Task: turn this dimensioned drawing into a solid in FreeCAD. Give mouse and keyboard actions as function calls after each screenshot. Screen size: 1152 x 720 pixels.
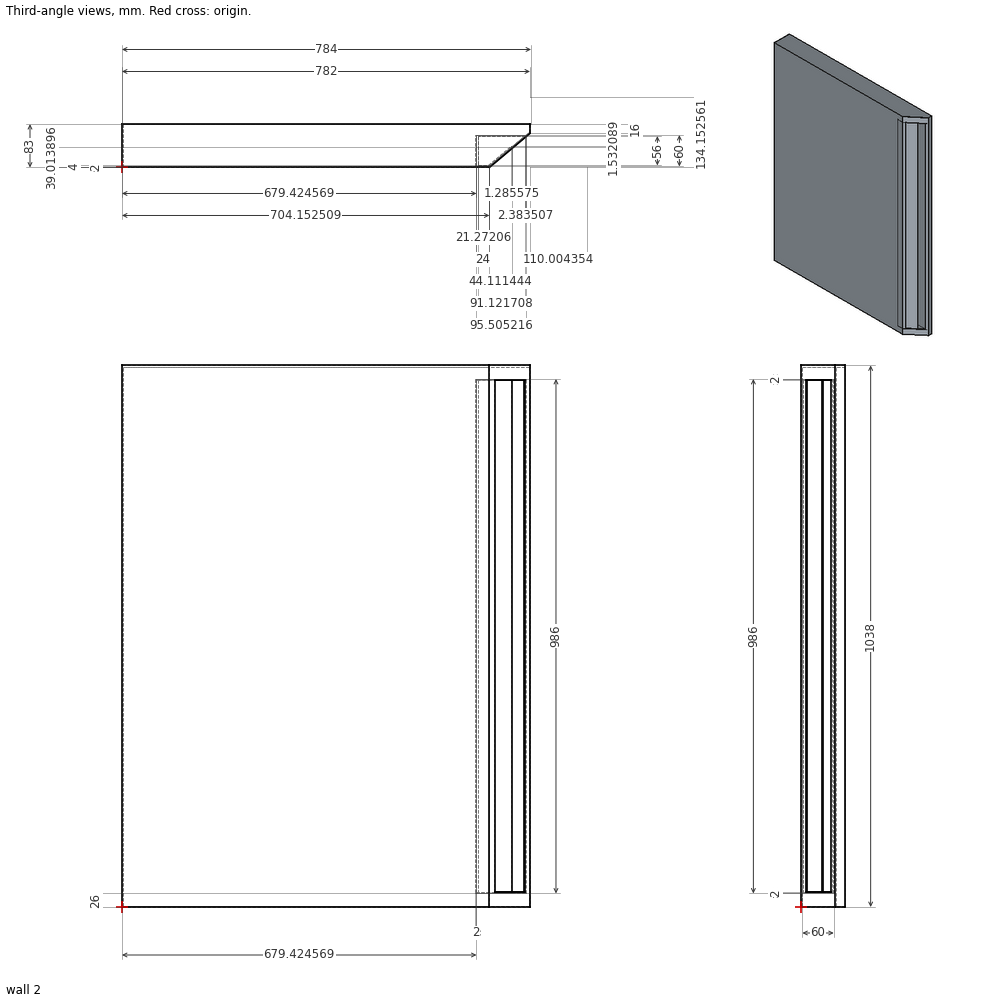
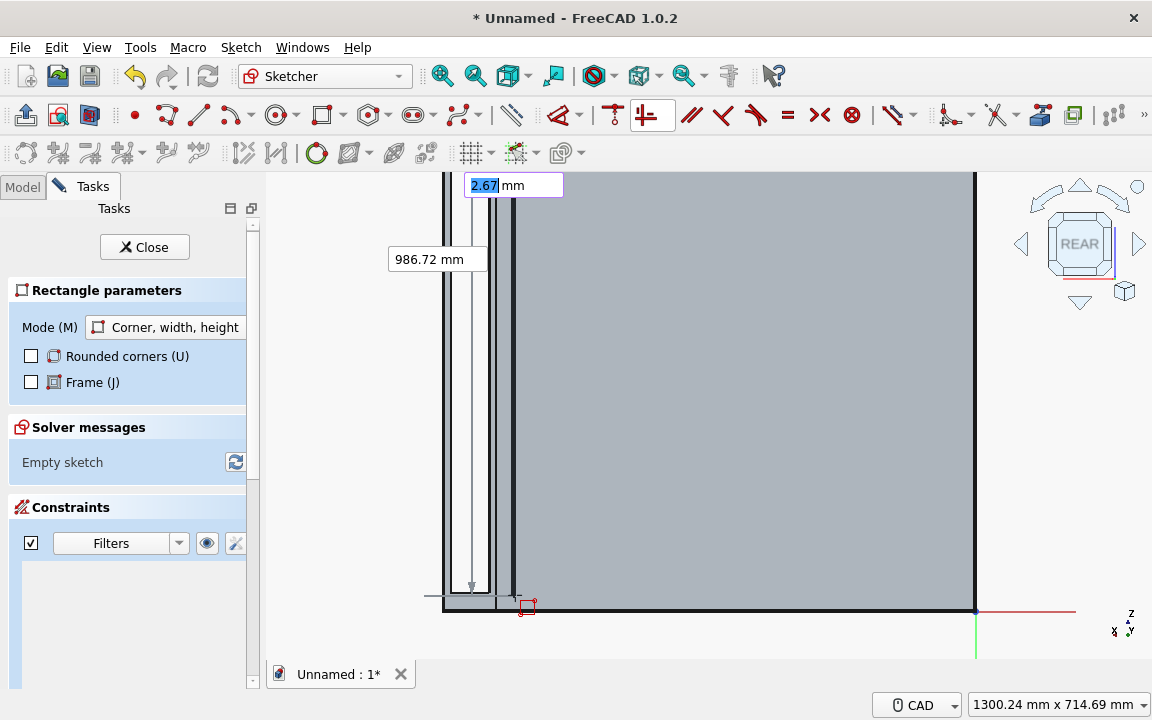
click(514, 594)
key(Escape)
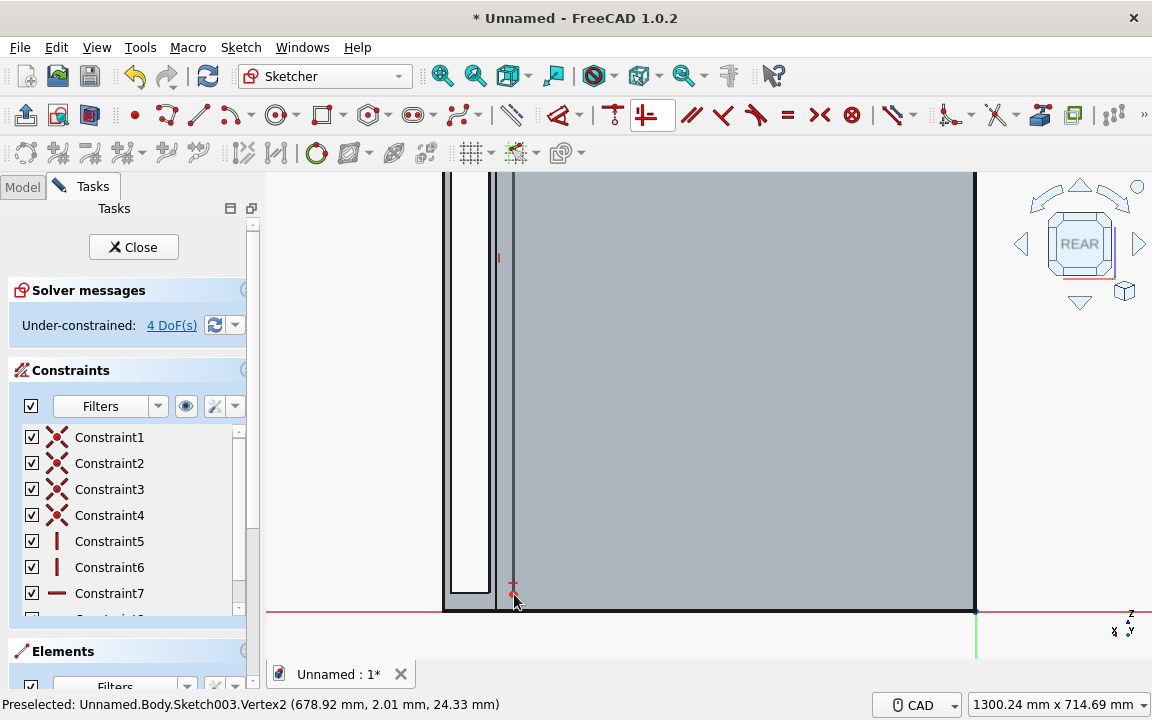
click(558, 116)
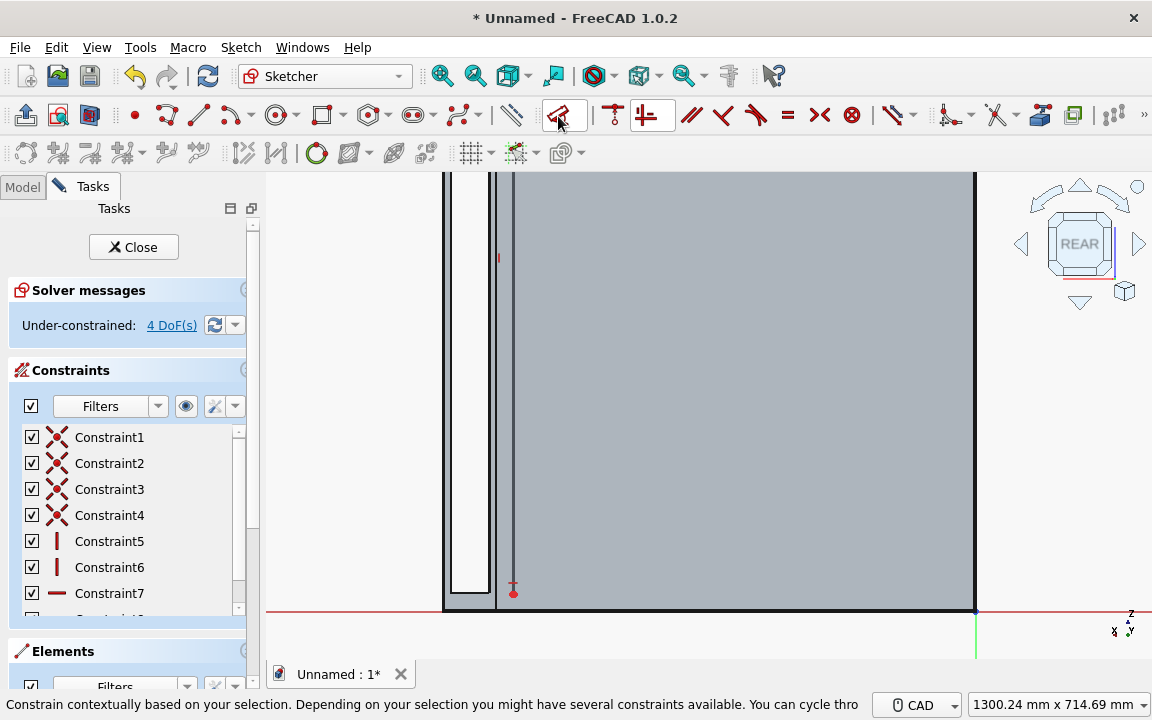
scroll(513, 595, up, 17)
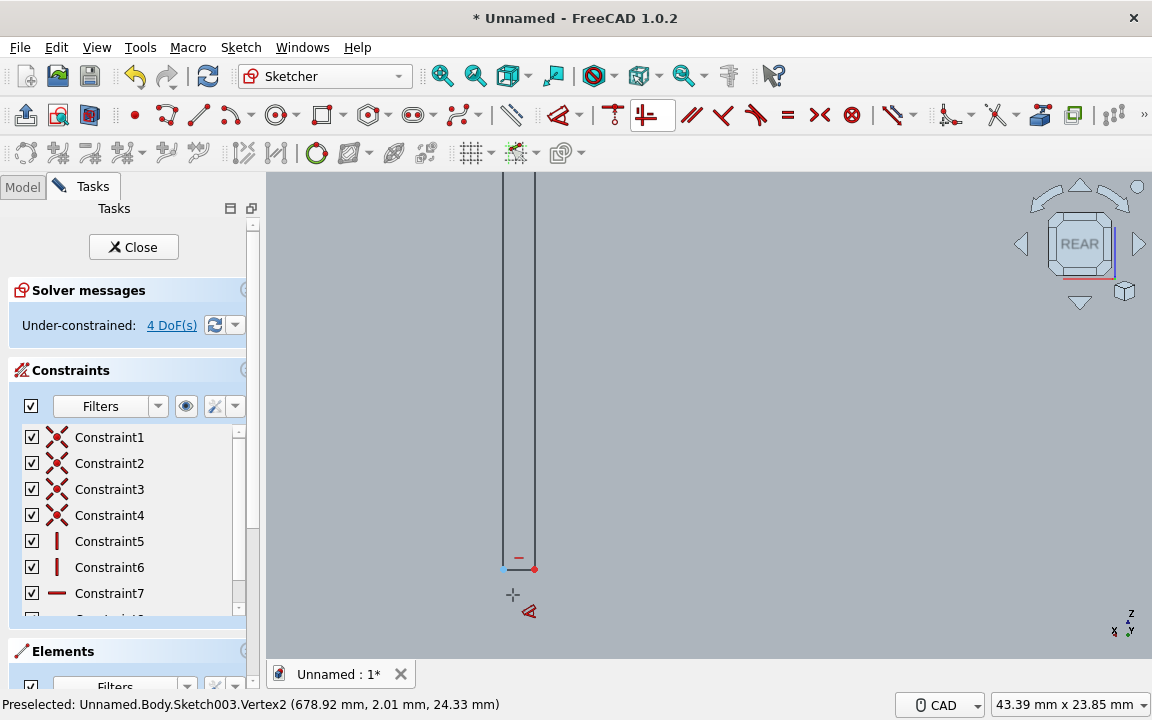
click(519, 570)
click(519, 604)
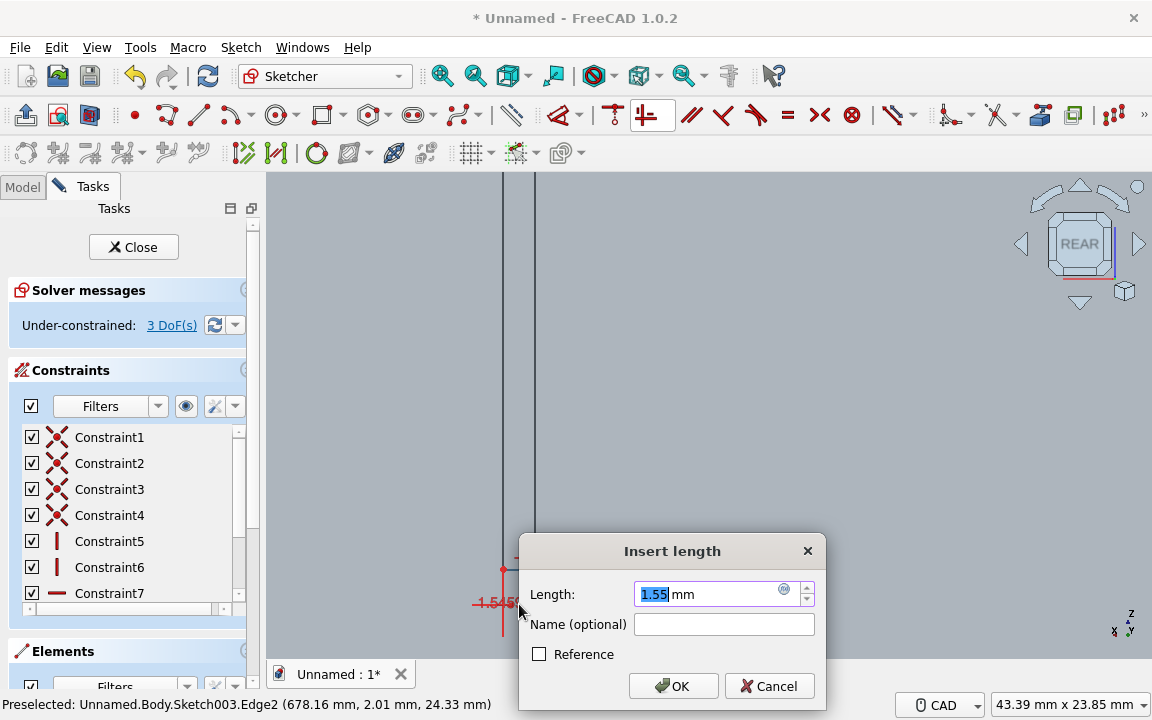
text(2)
key(Return)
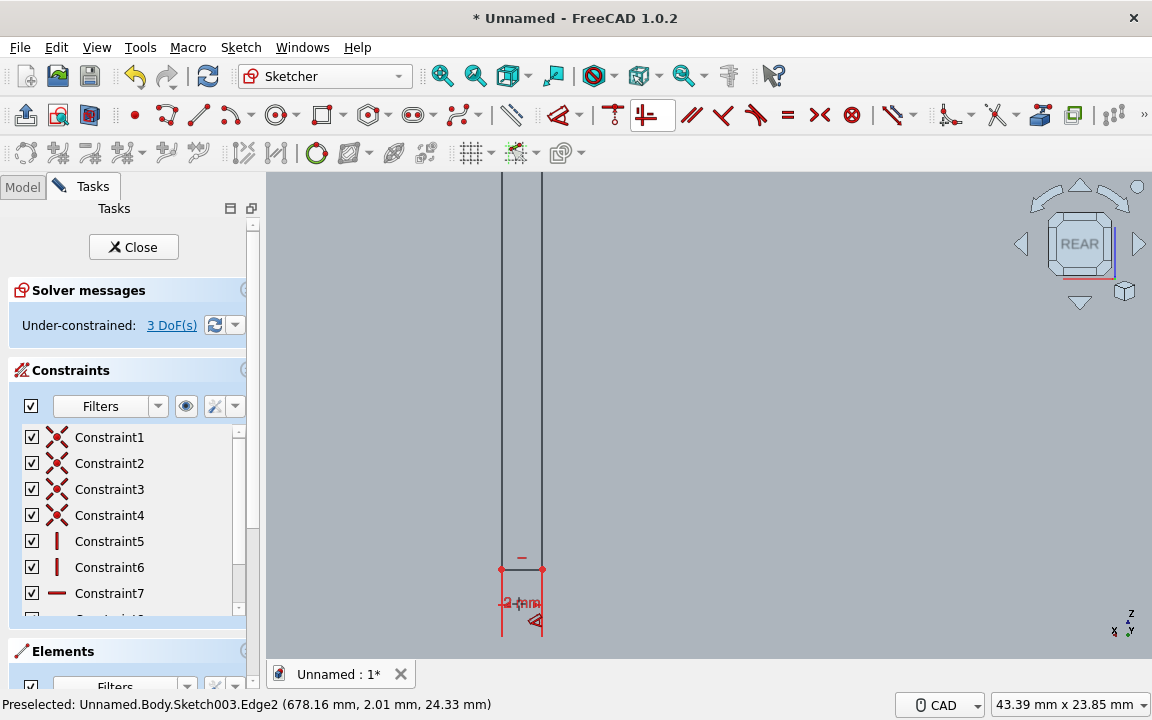
scroll(640, 416, down, 15)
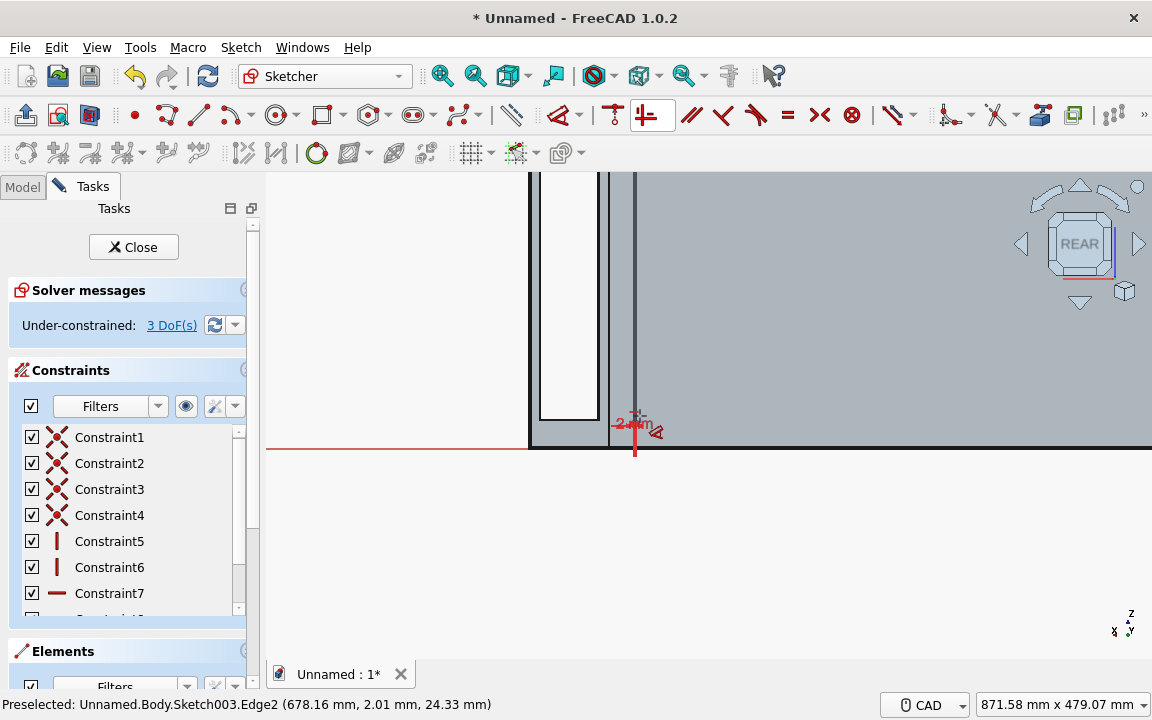
scroll(495, 623, down, 6)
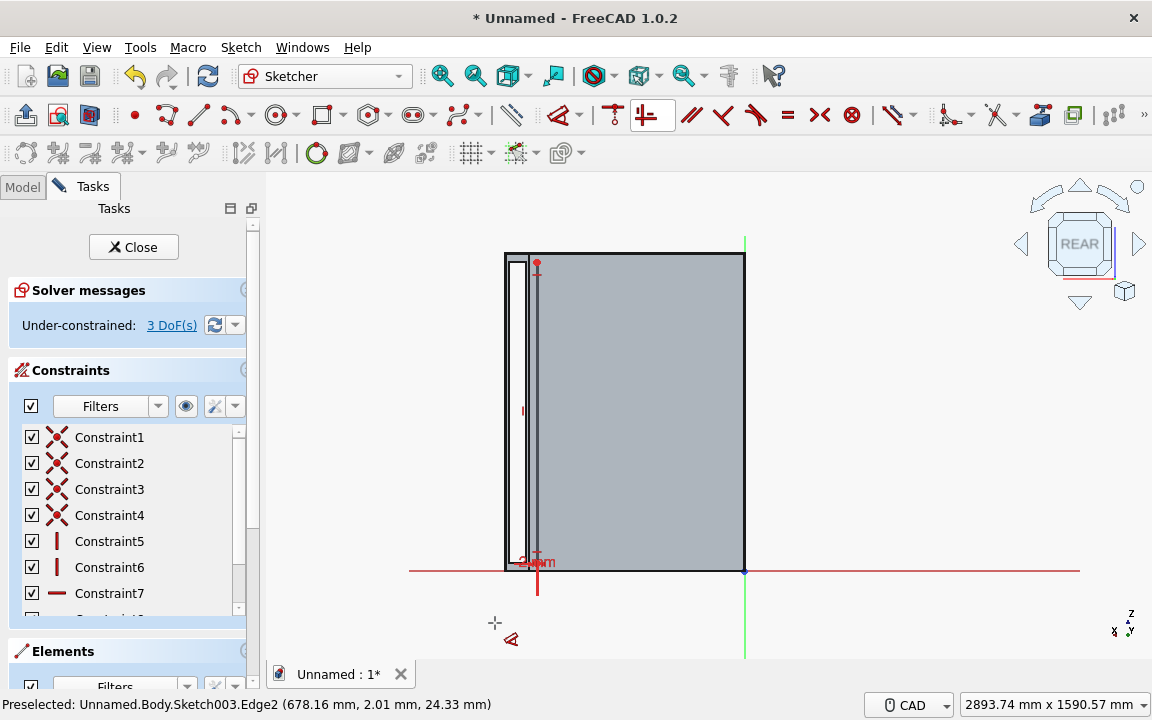
scroll(537, 353, up, 14)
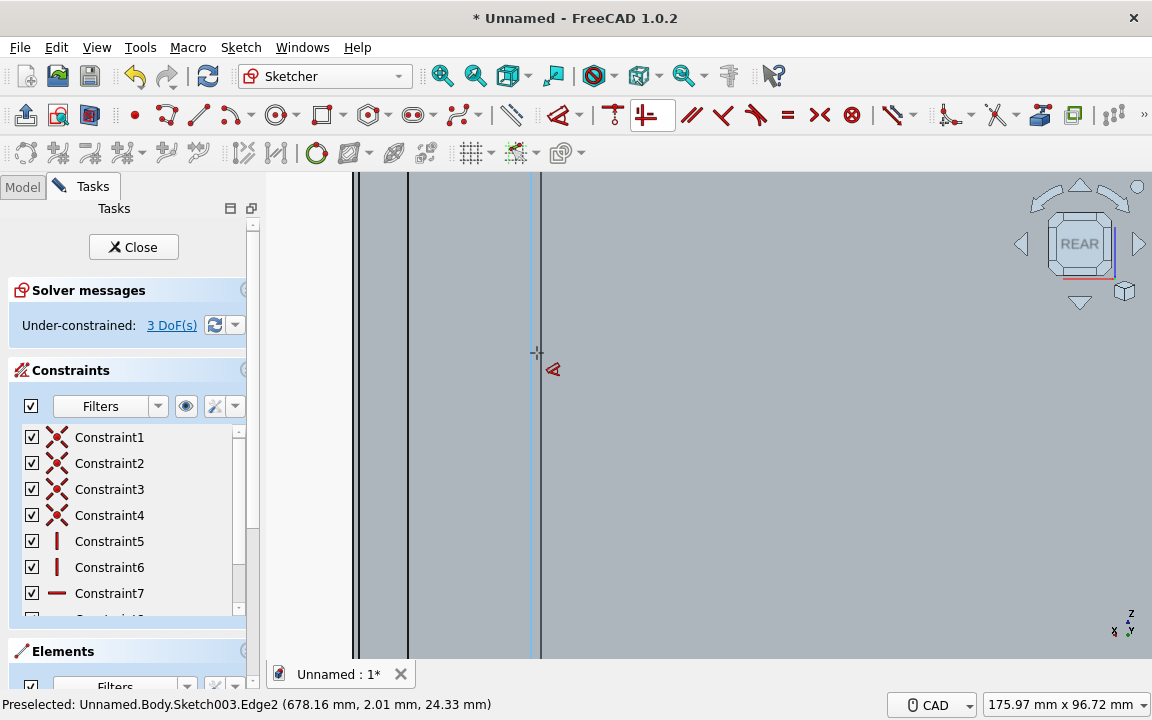
click(531, 341)
click(497, 416)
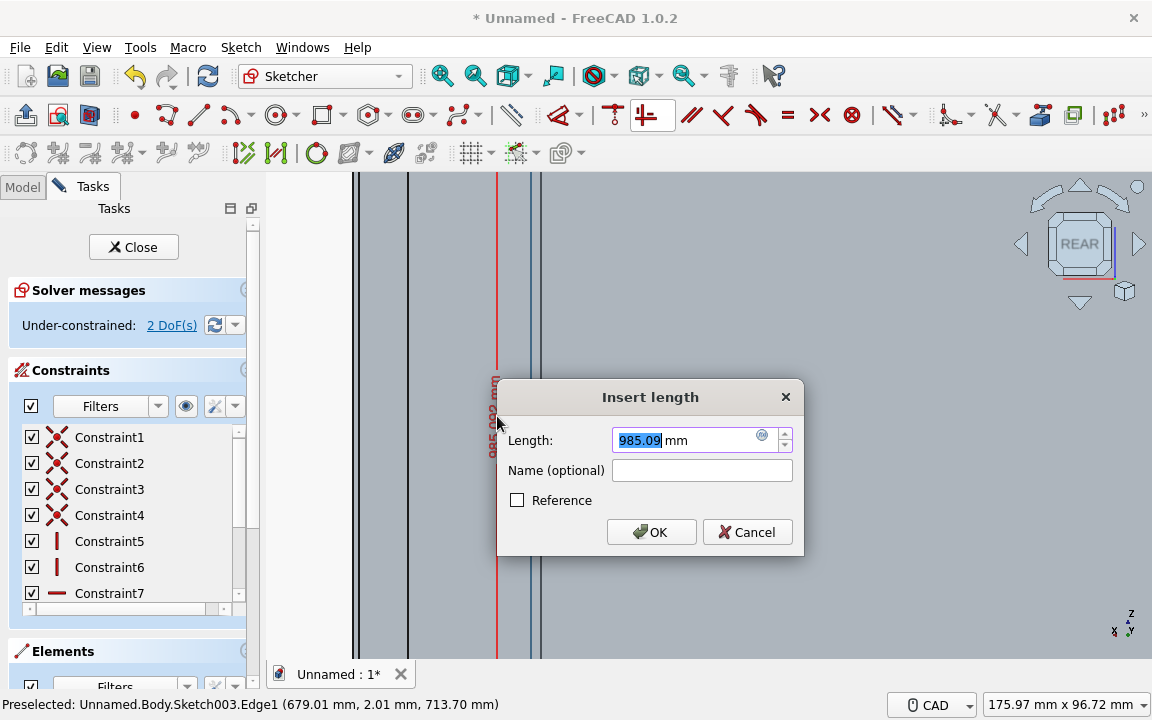
text(986)
key(Return)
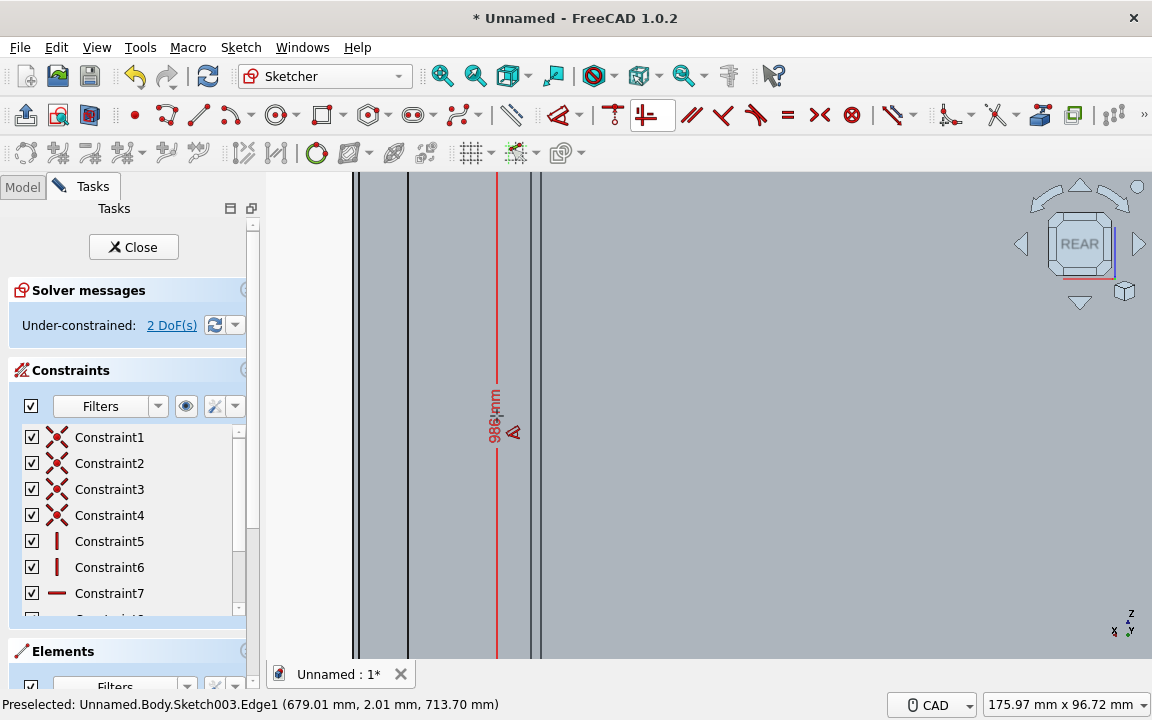
scroll(537, 353, down, 14)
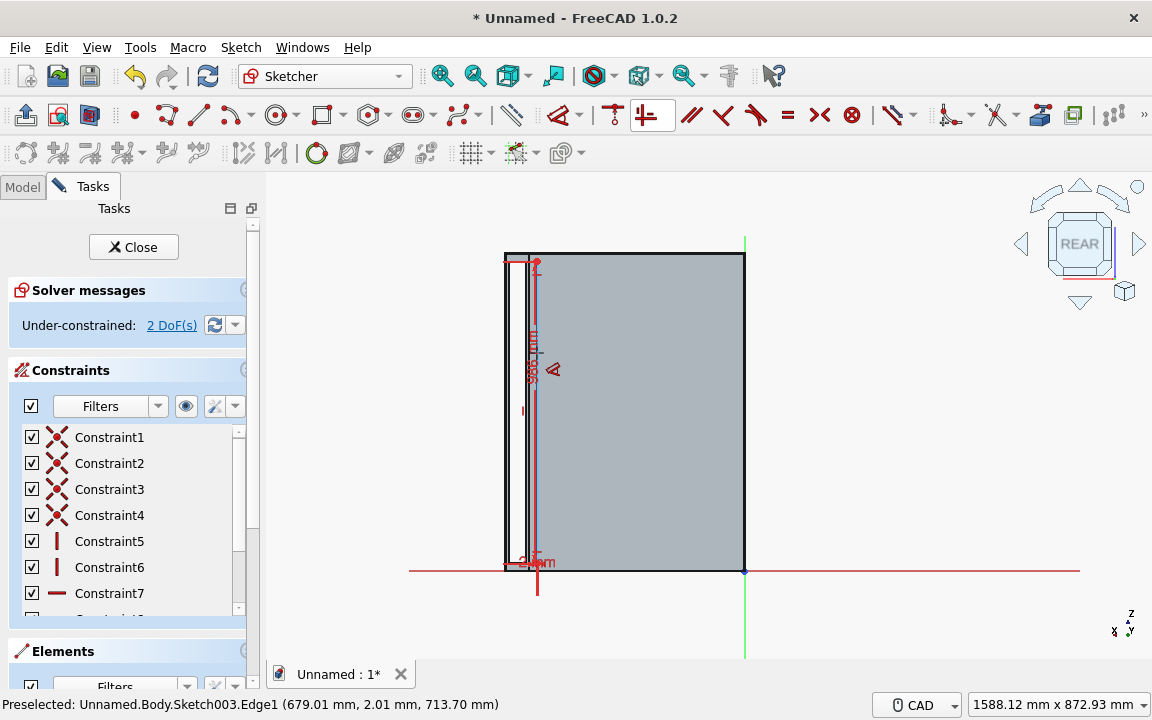
scroll(537, 564, up, 14)